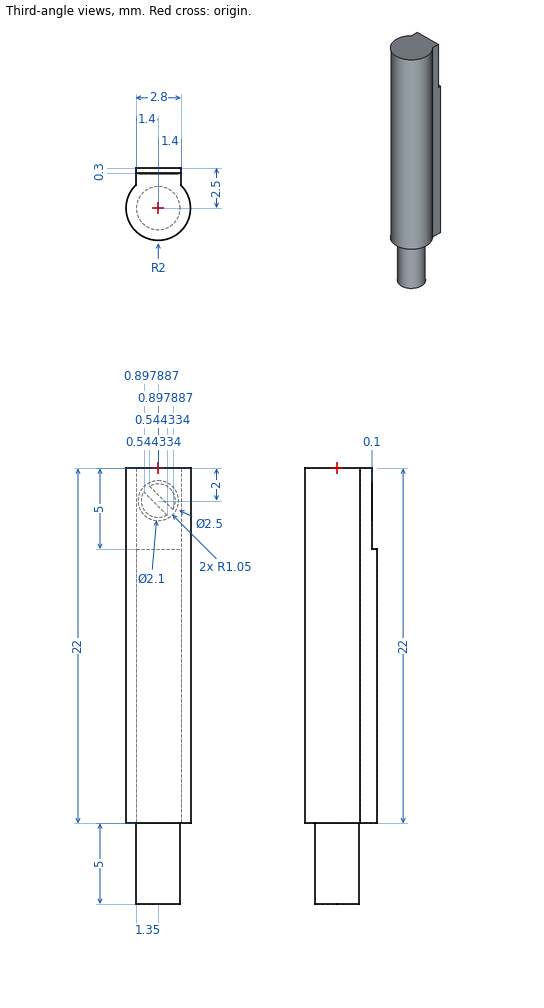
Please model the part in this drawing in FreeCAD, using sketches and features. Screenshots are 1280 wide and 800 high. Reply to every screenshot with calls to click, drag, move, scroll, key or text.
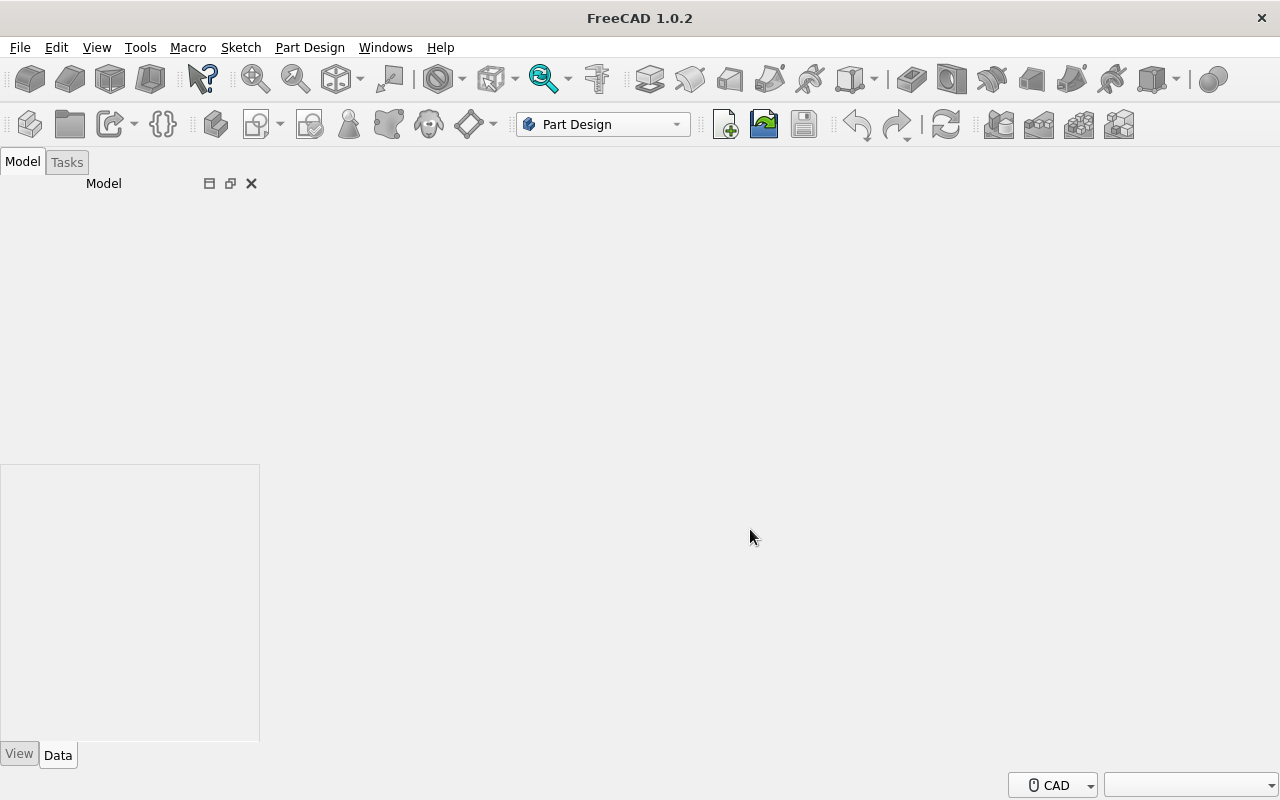
click(724, 124)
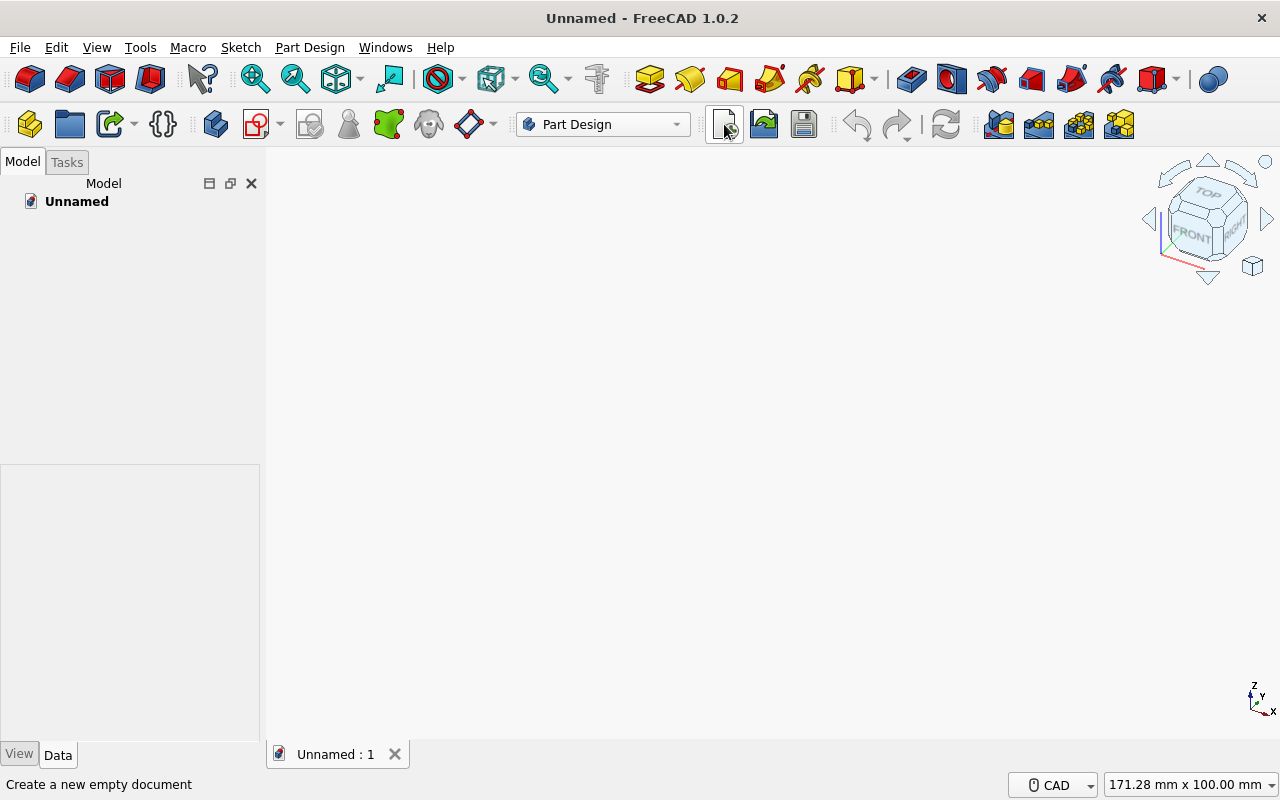
click(256, 124)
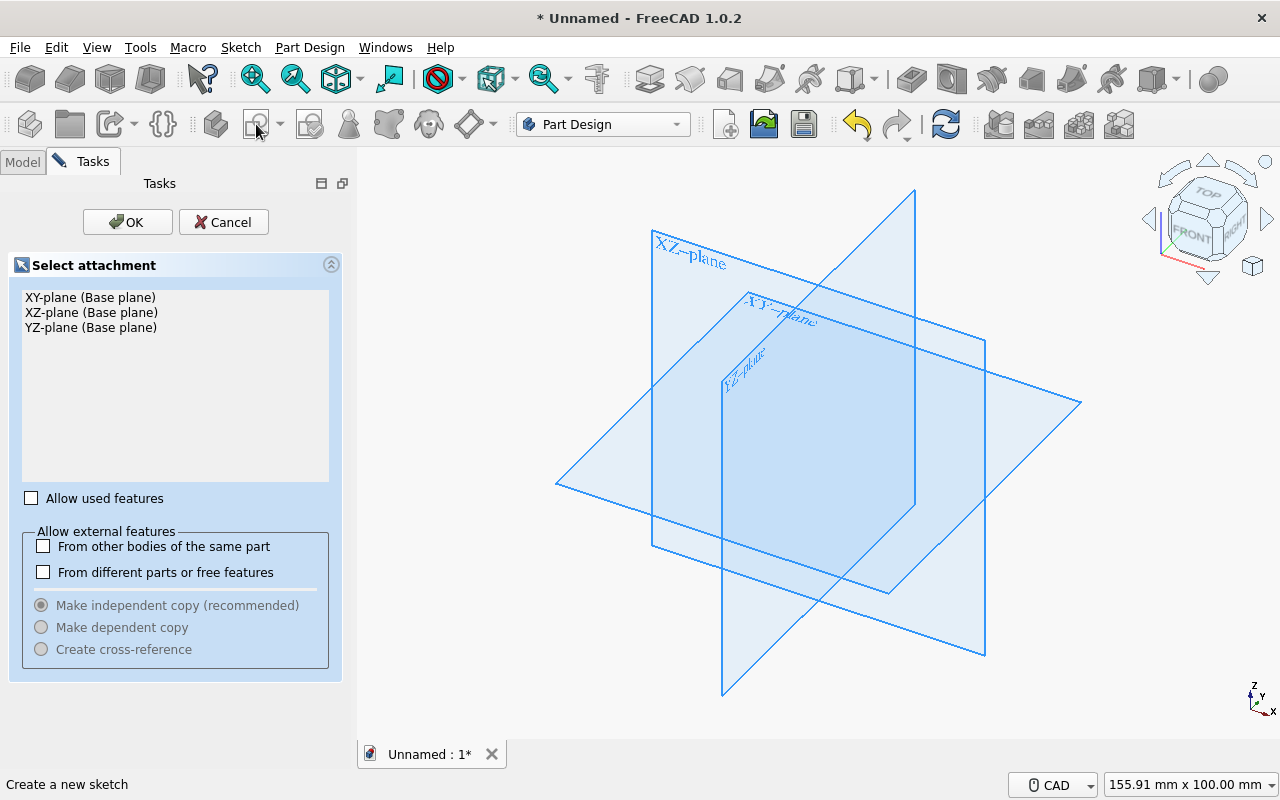
click(82, 298)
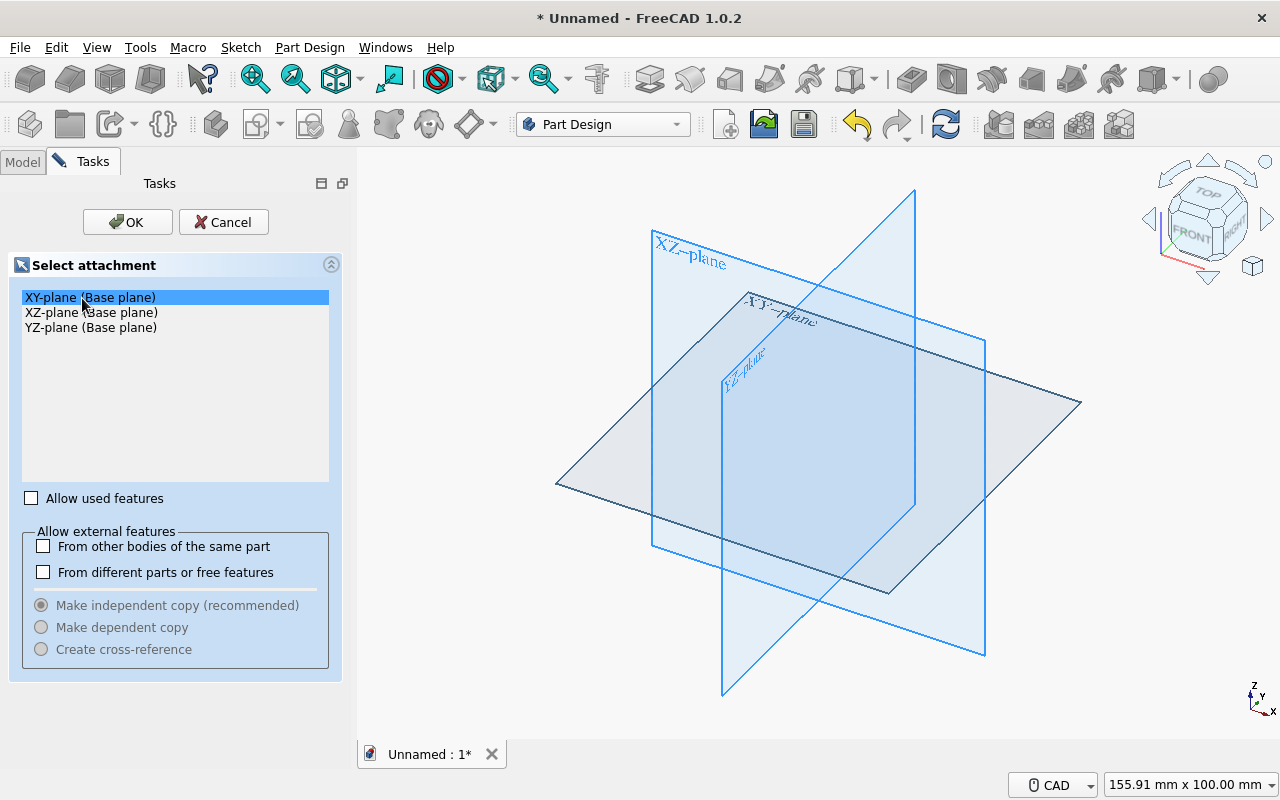
click(128, 222)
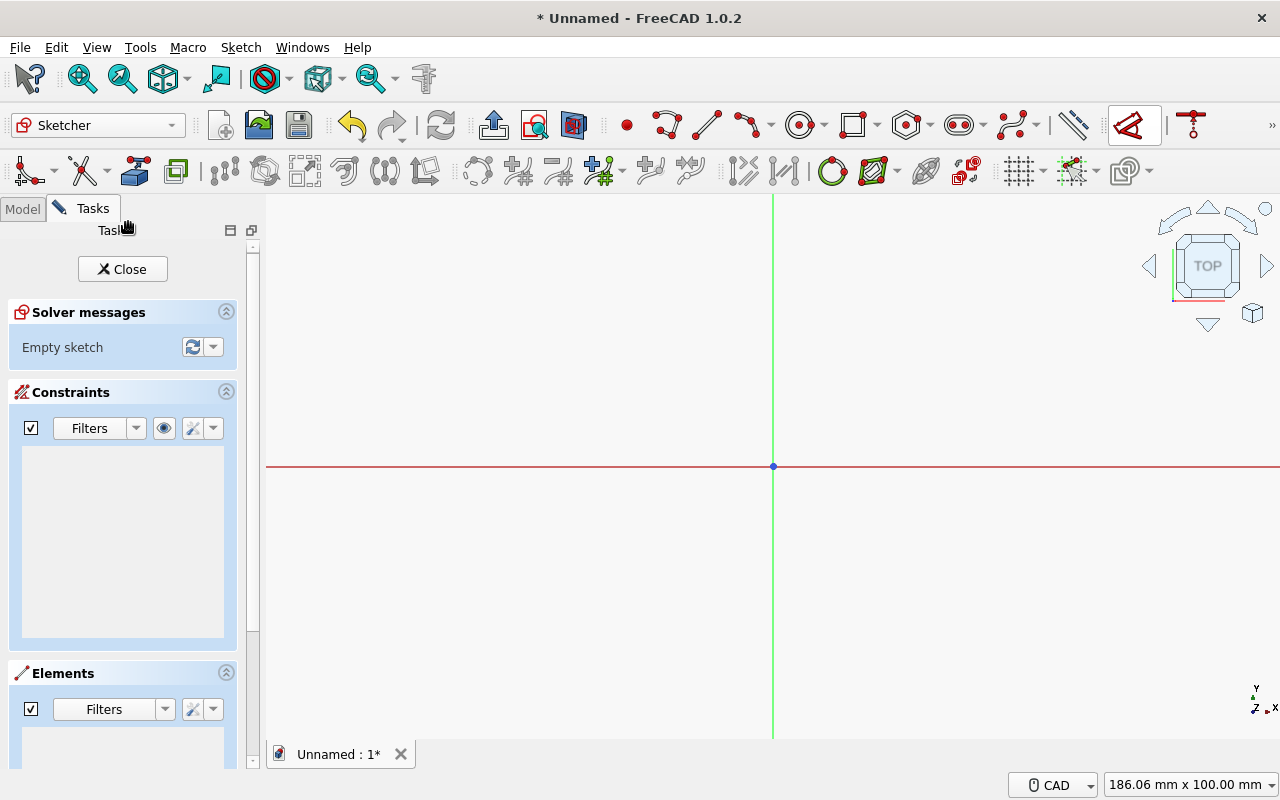
scroll(778, 465, up, 13)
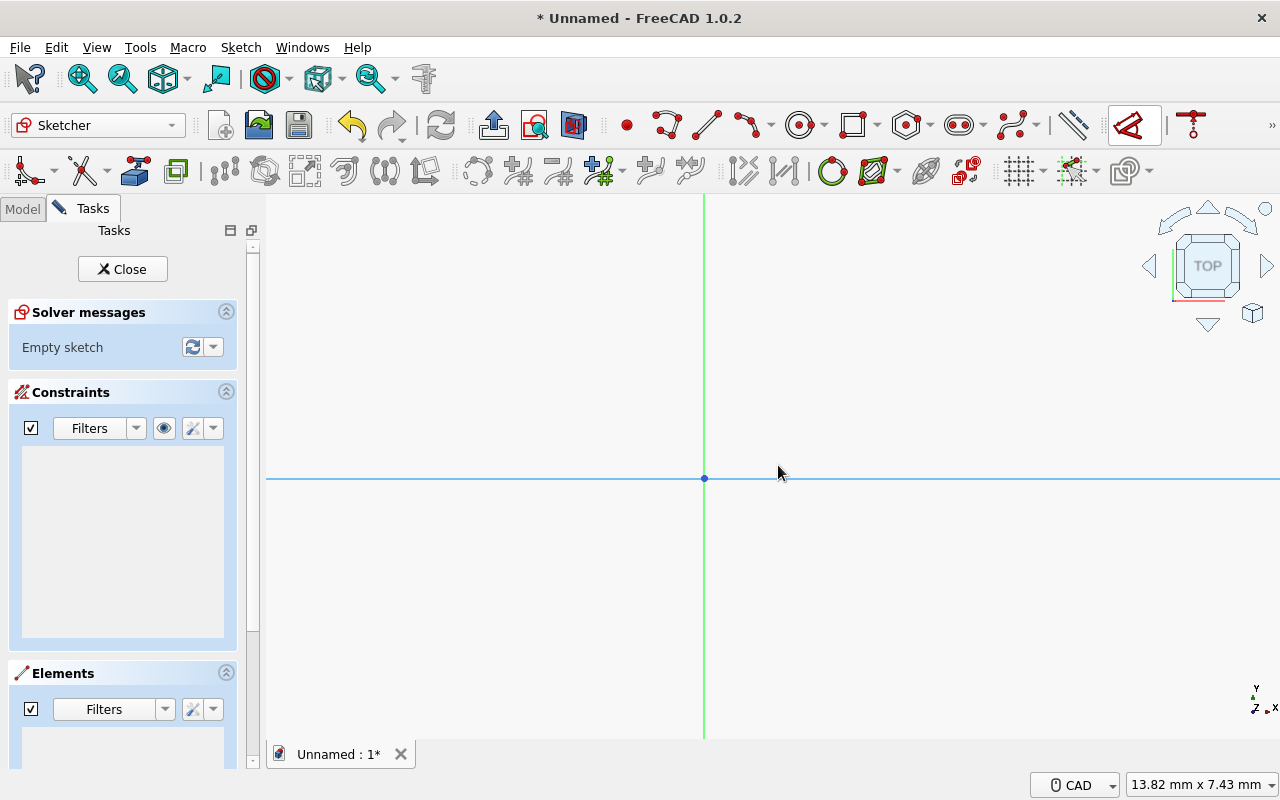
click(668, 126)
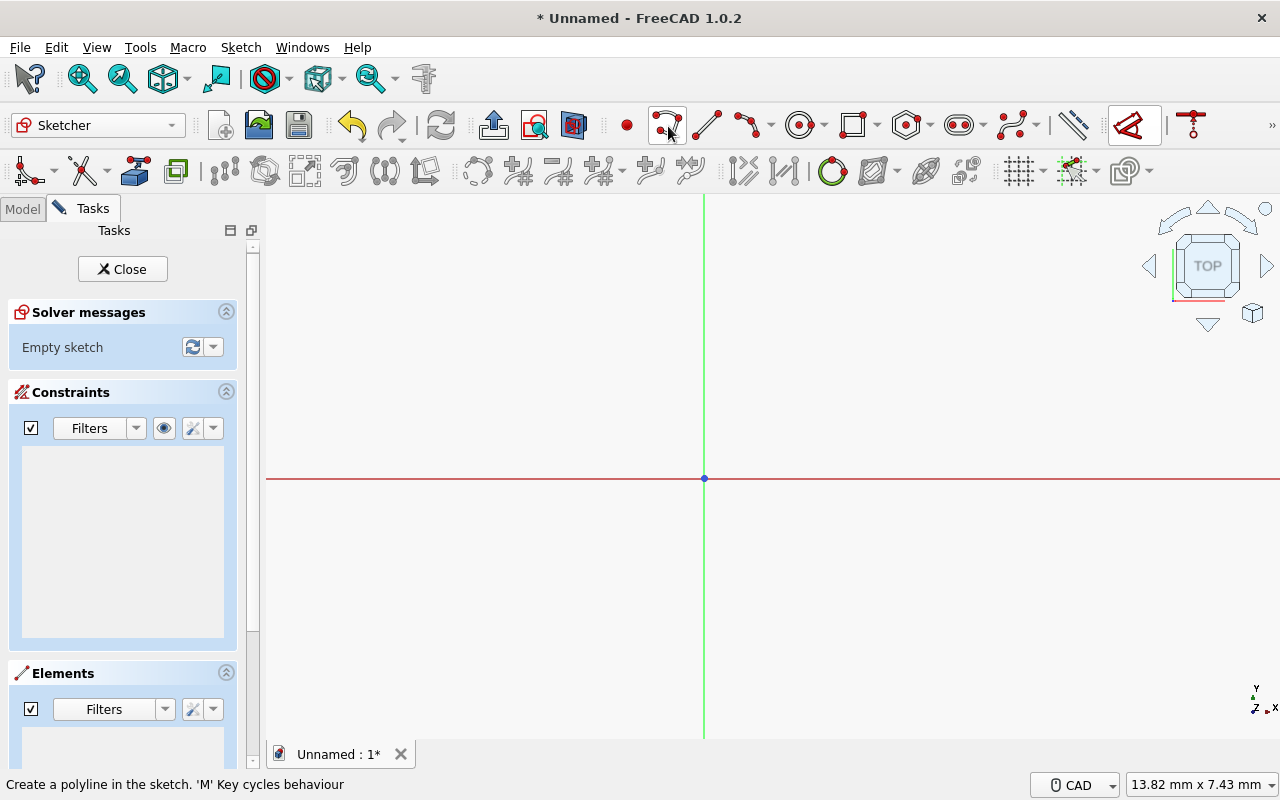
click(807, 374)
click(807, 296)
click(602, 296)
click(602, 374)
right_click(602, 374)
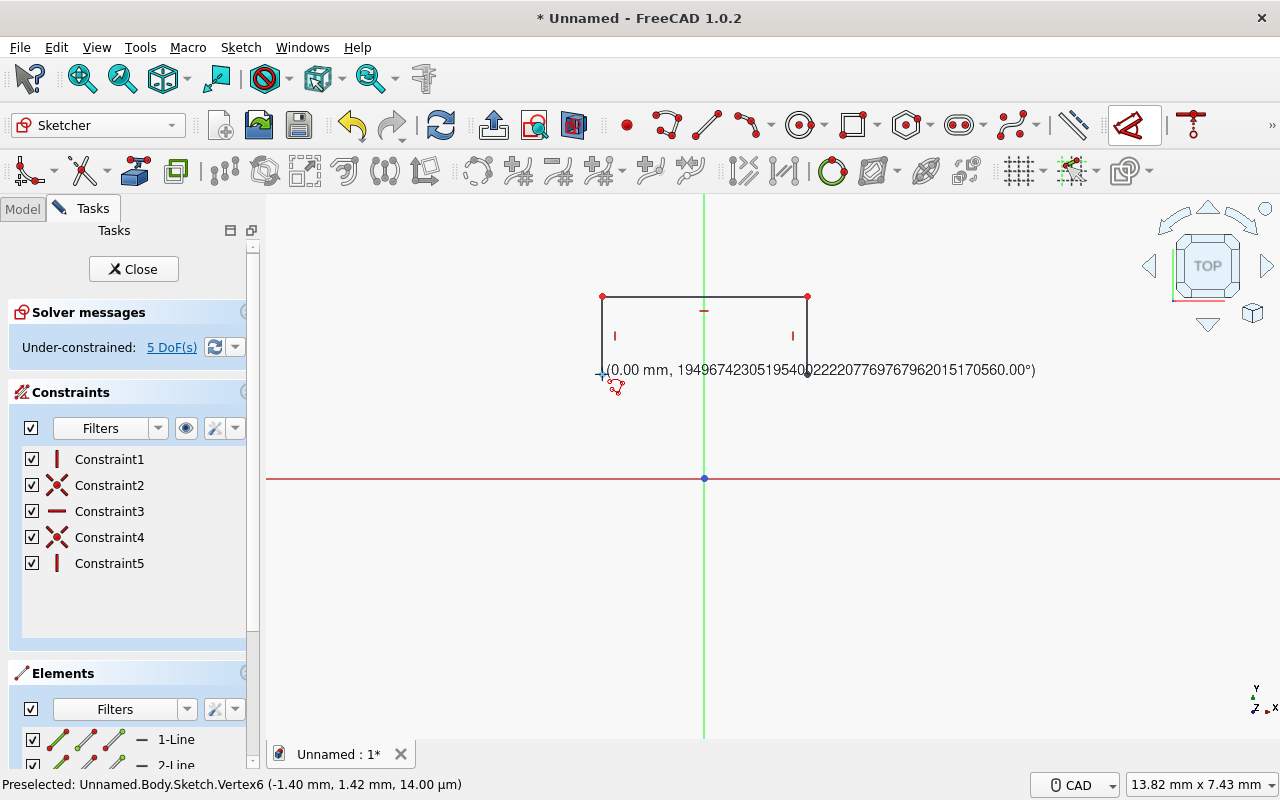
click(748, 126)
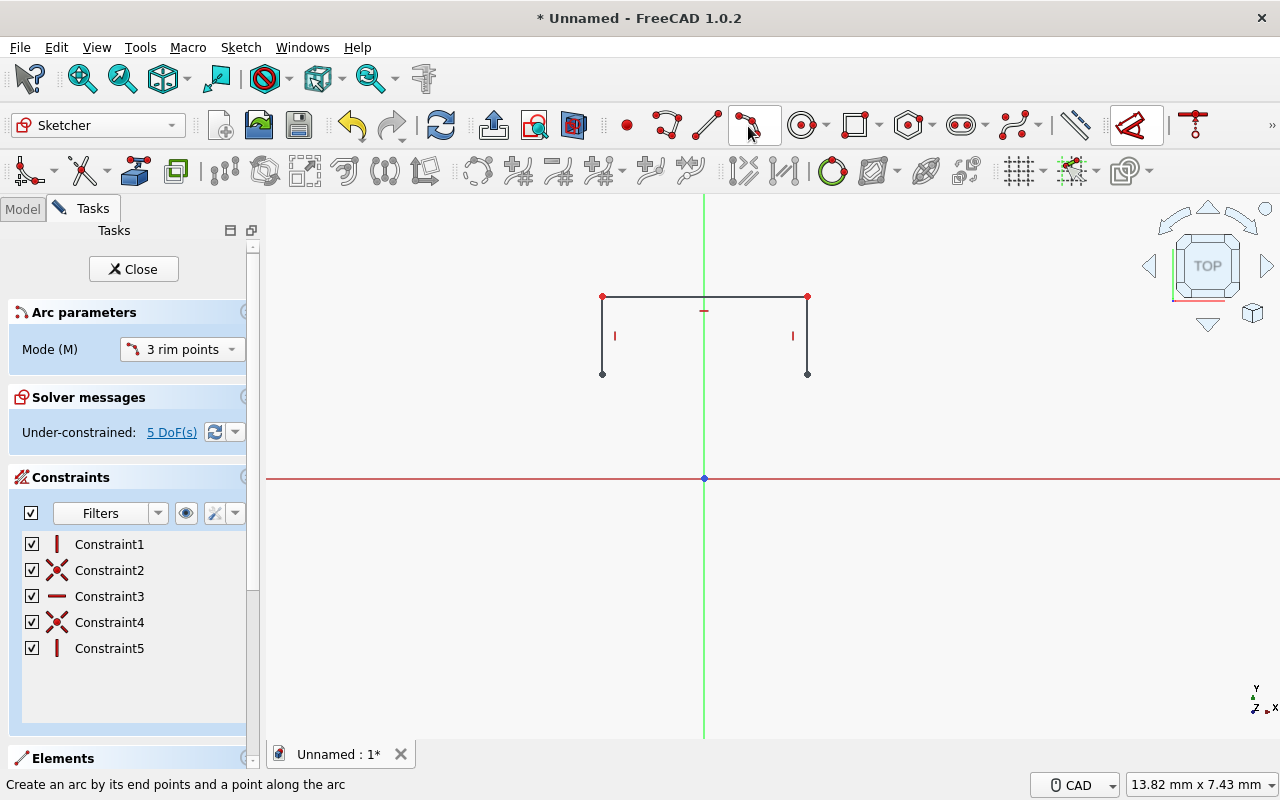
click(602, 375)
click(807, 375)
click(637, 610)
key(Escape)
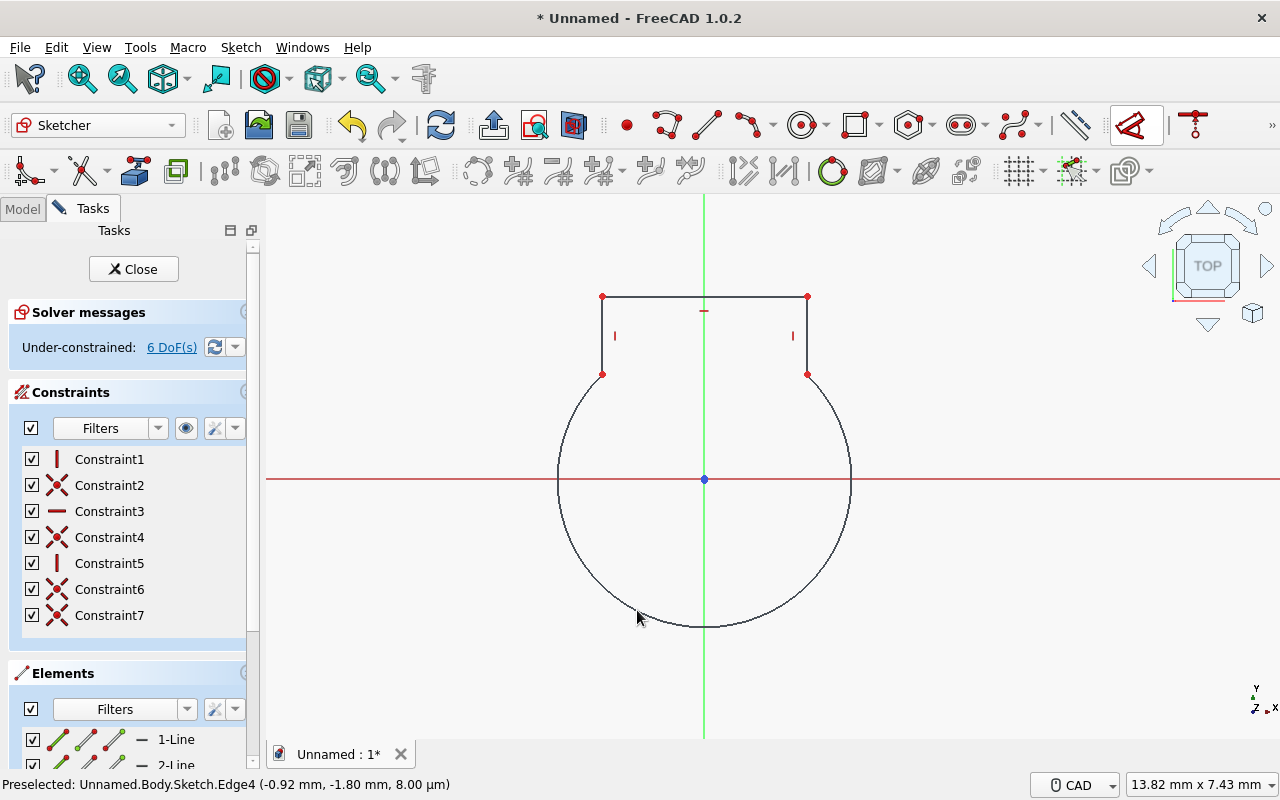
drag(694, 469, 714, 490)